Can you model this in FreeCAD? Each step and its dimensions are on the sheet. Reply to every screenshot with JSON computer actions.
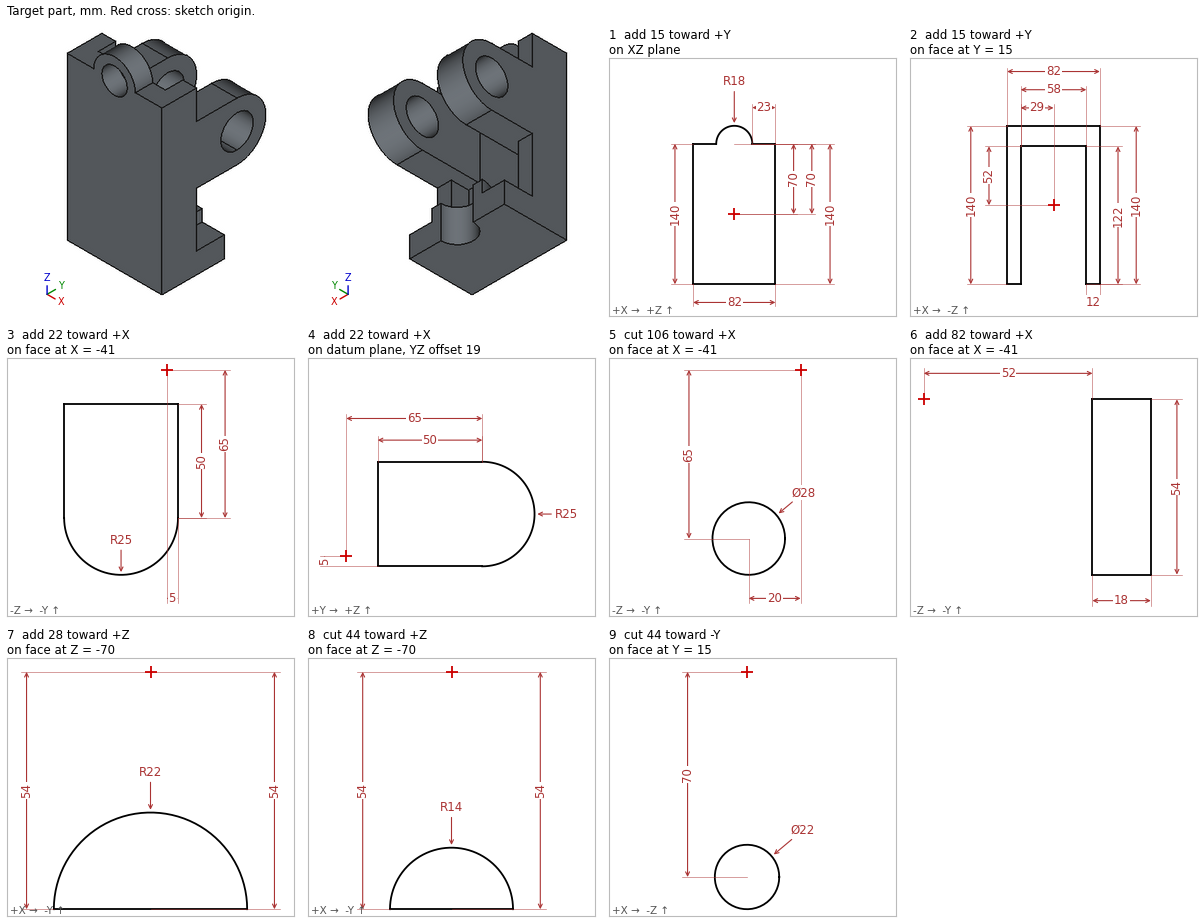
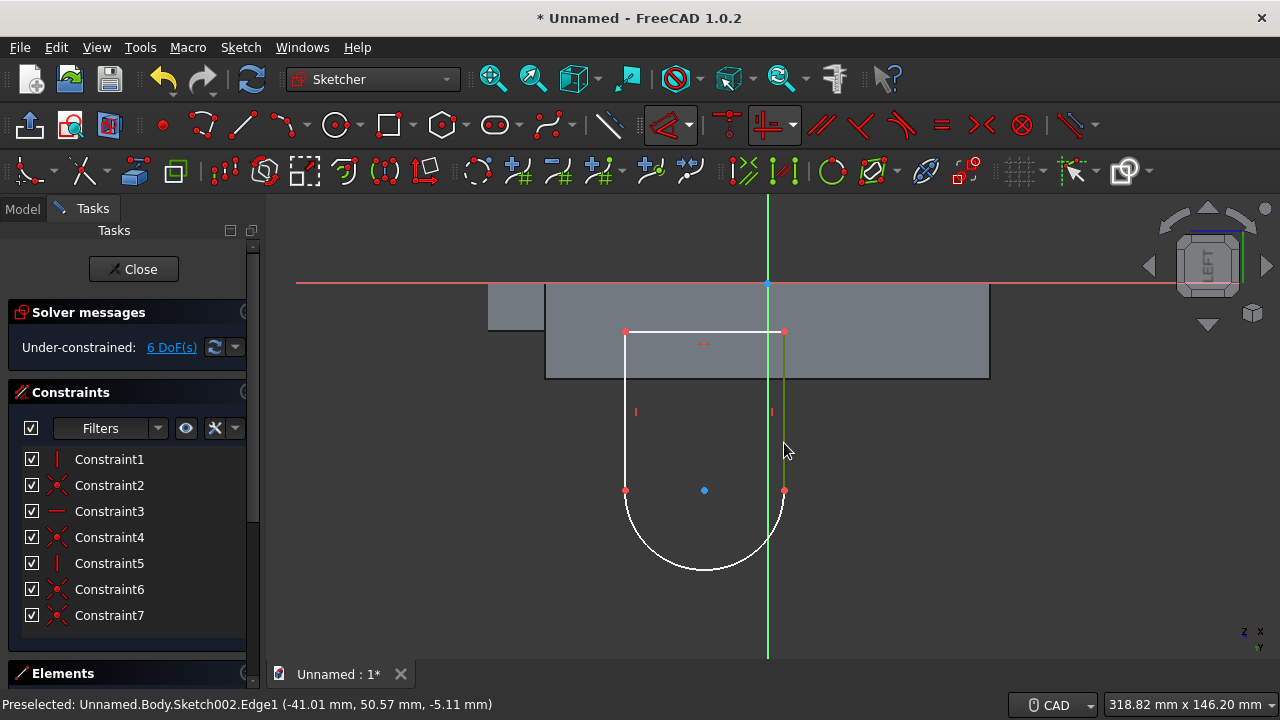
{"action": "left_click", "coordinate": [658, 555]}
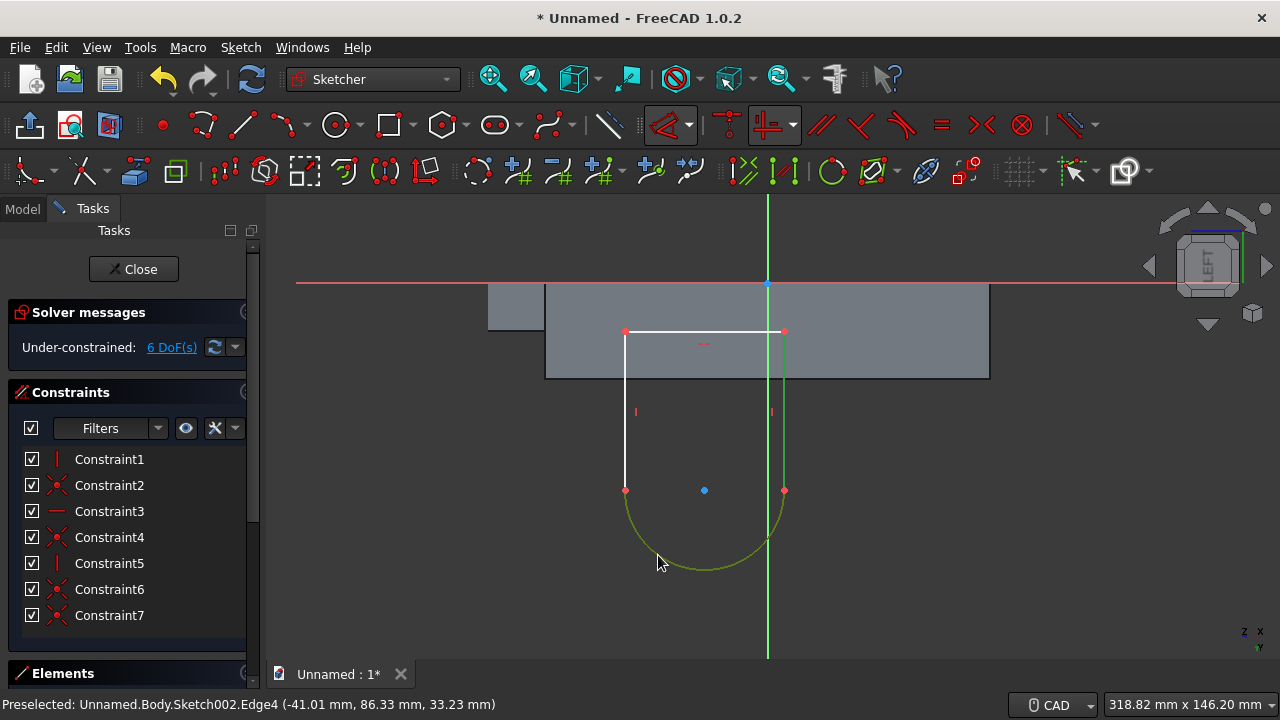
{"action": "key", "text": "t"}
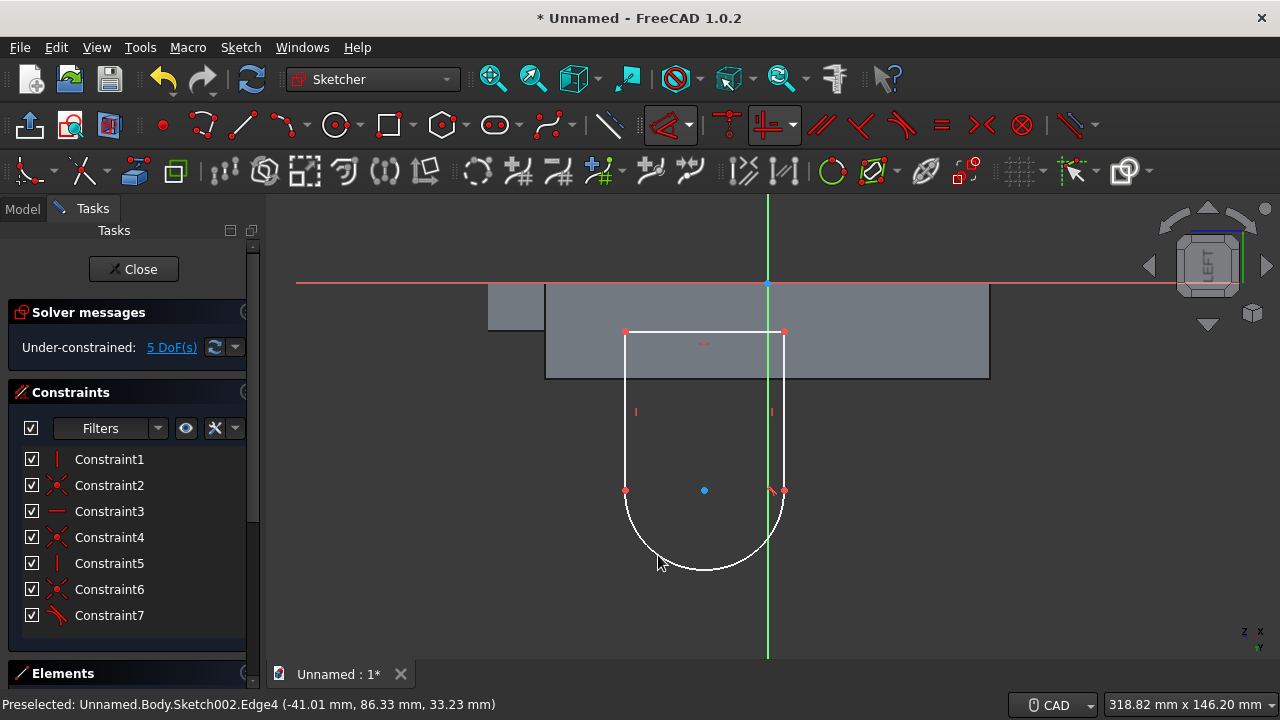
{"action": "left_click", "coordinate": [625, 380]}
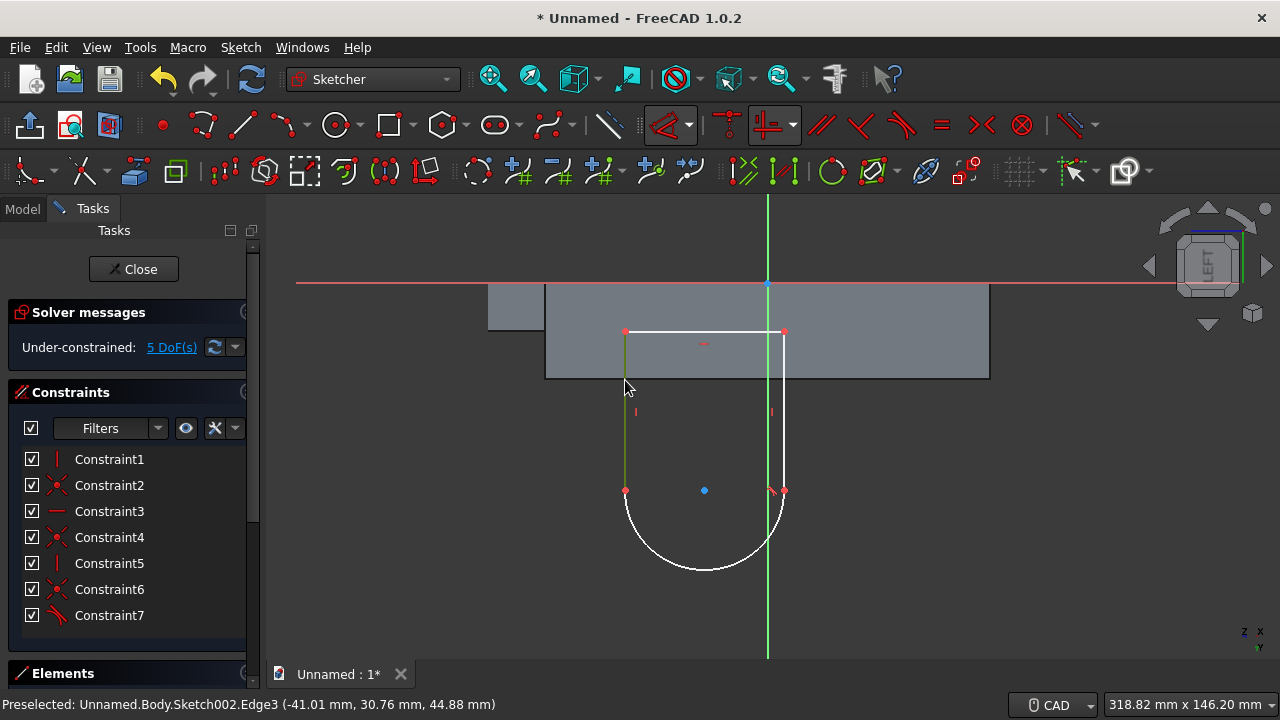
{"action": "left_click", "coordinate": [658, 555]}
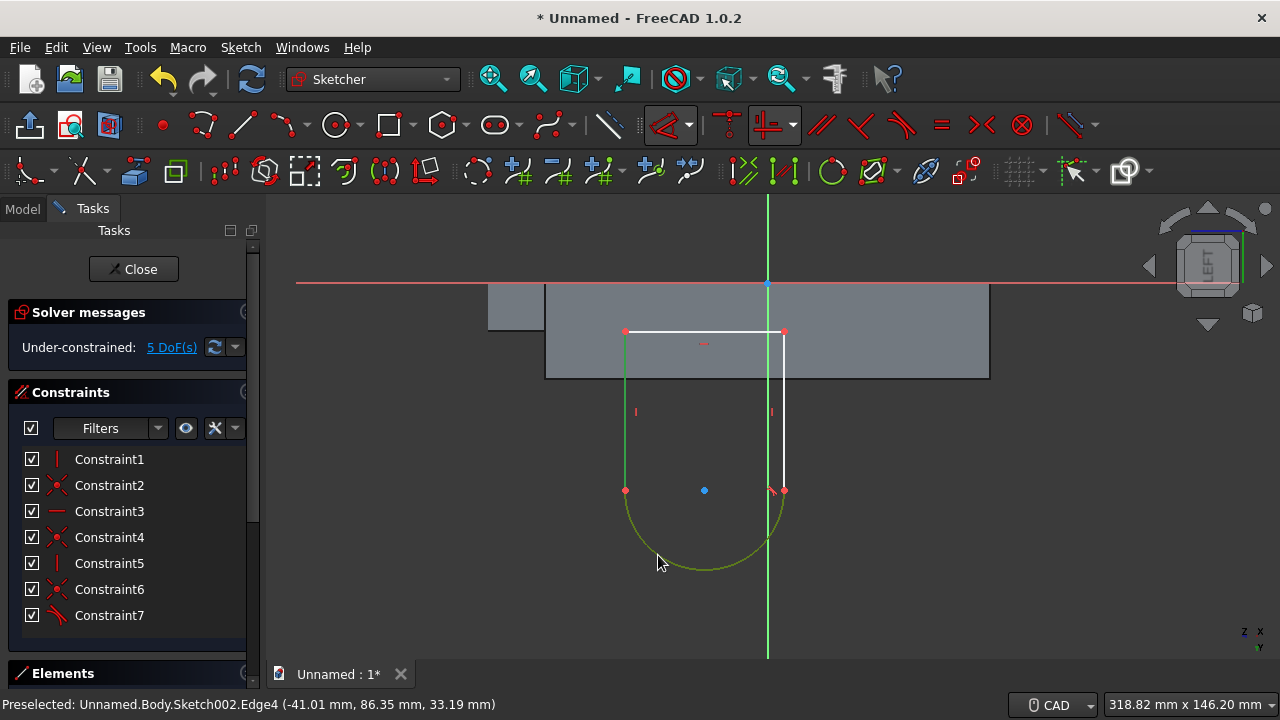
{"action": "key", "text": "t"}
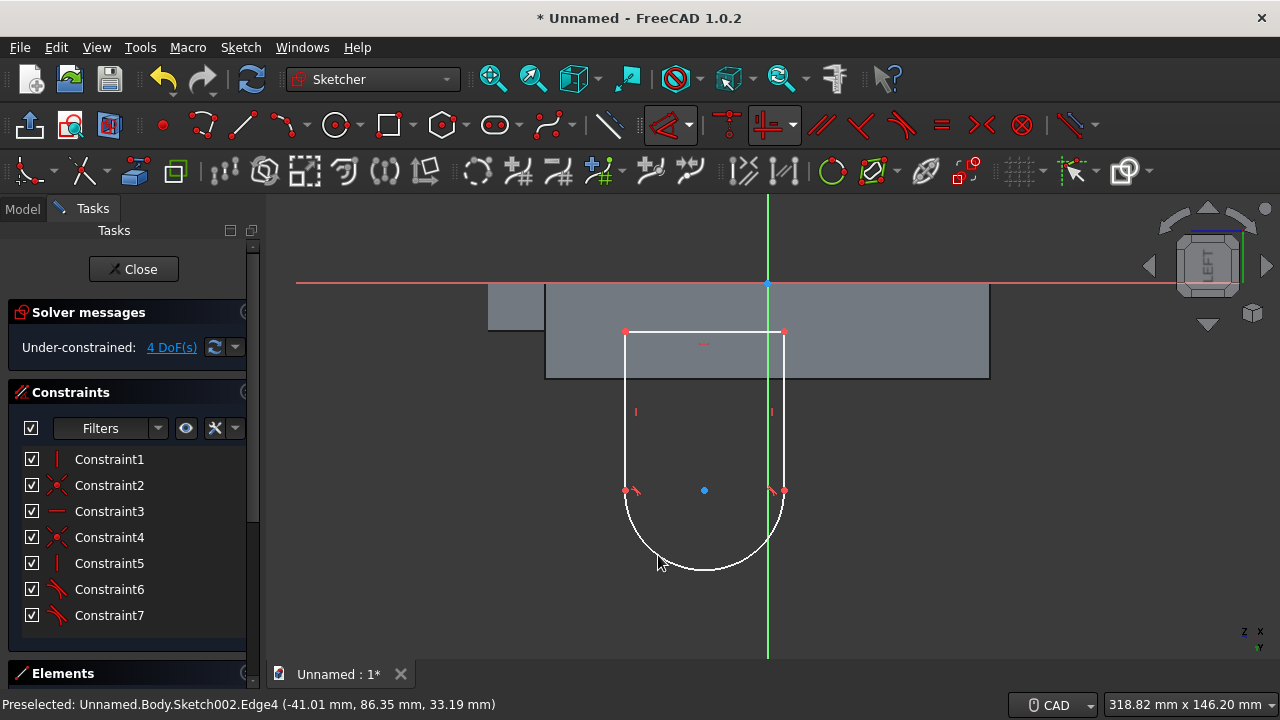
{"action": "left_click", "coordinate": [658, 555]}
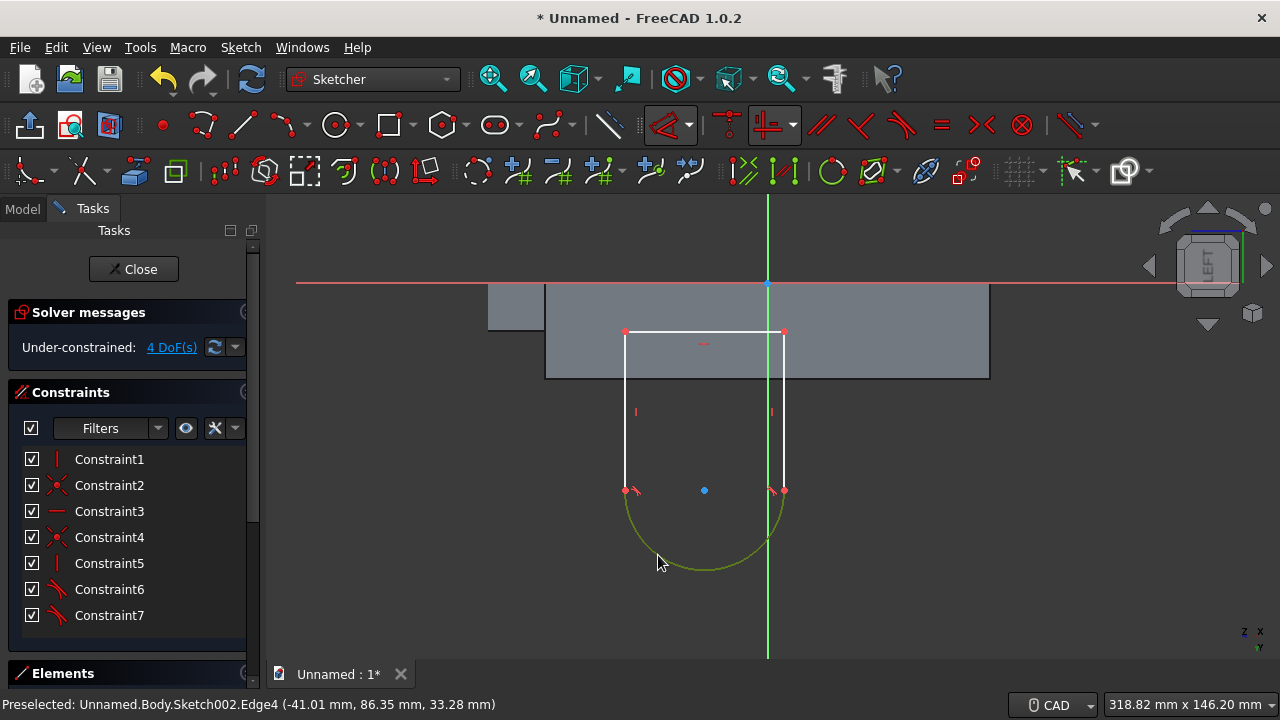
{"action": "key", "text": "k r"}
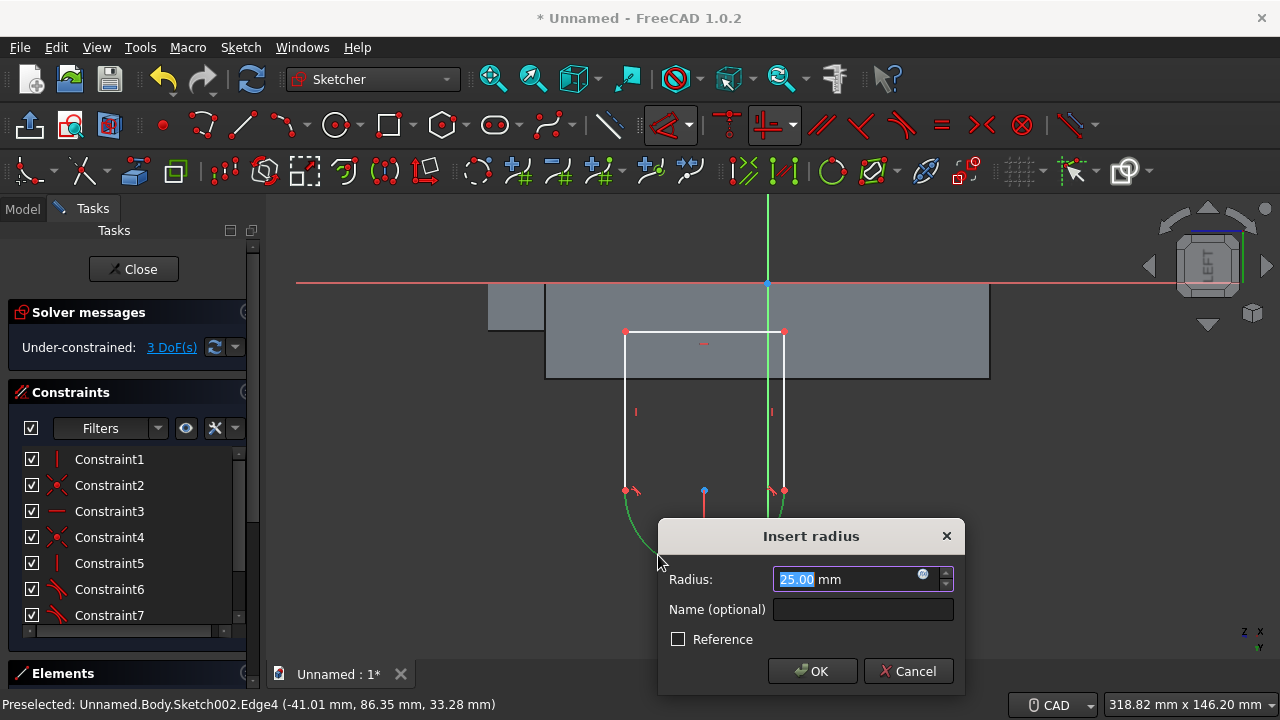
{"action": "type", "text": "25"}
{"action": "key", "text": "Return"}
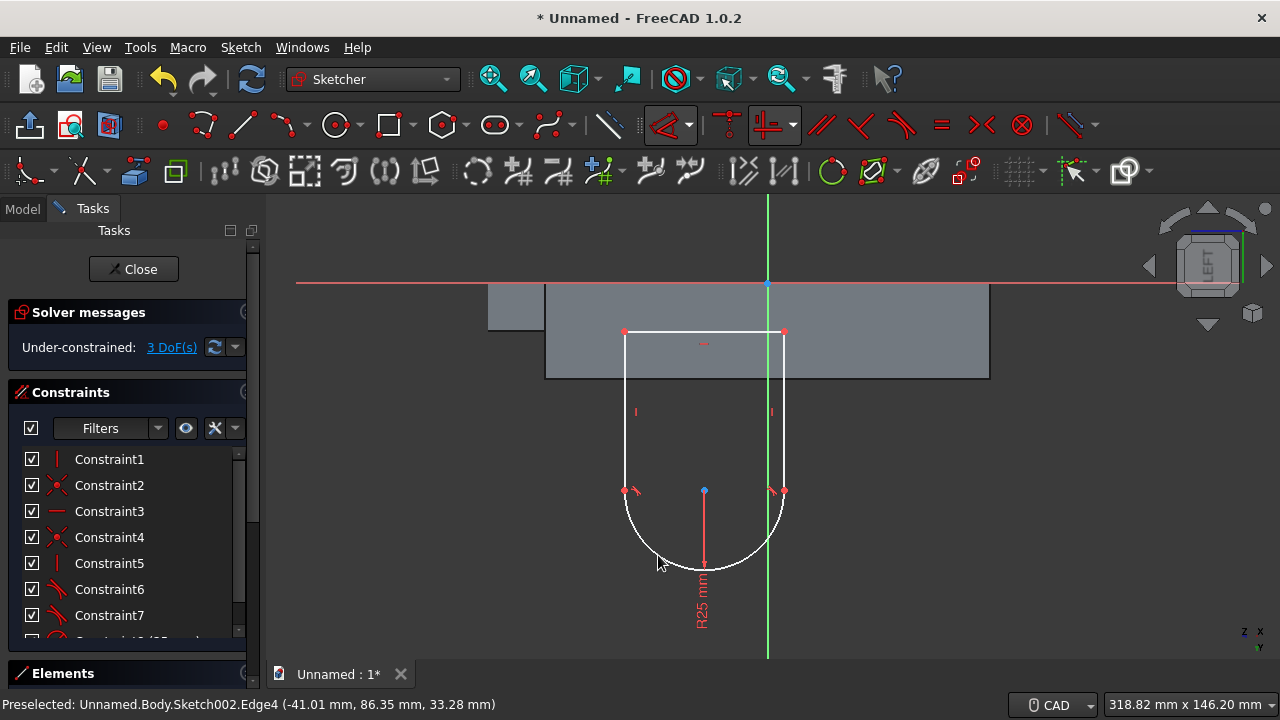
{"action": "left_click", "coordinate": [784, 443]}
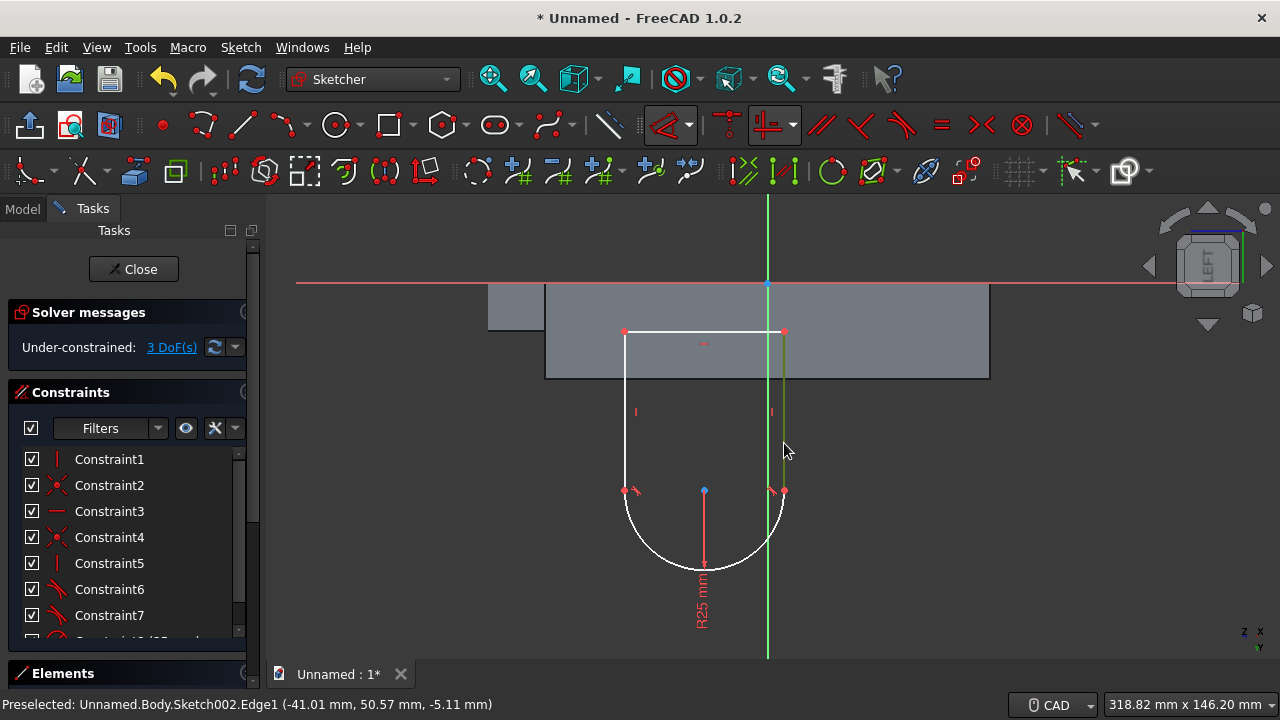
{"action": "key", "text": "i"}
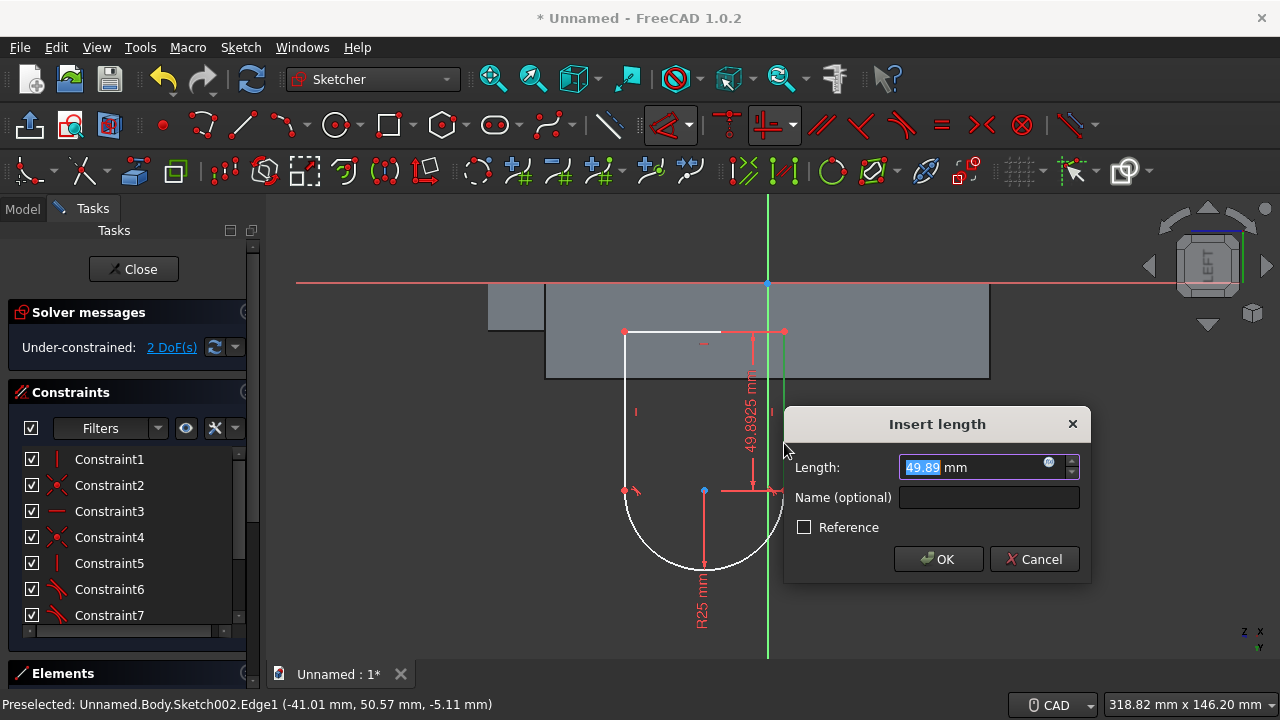
{"action": "type", "text": "50"}
{"action": "key", "text": "Return"}